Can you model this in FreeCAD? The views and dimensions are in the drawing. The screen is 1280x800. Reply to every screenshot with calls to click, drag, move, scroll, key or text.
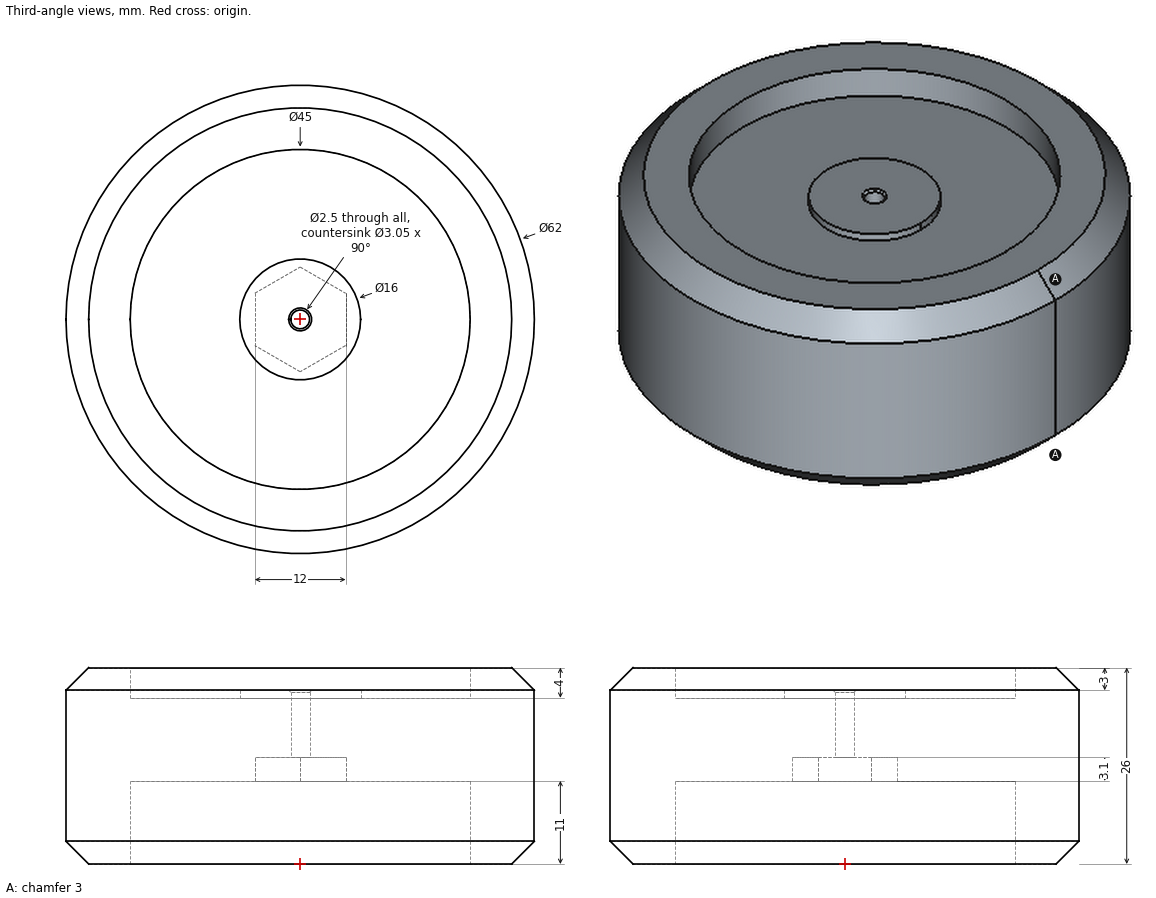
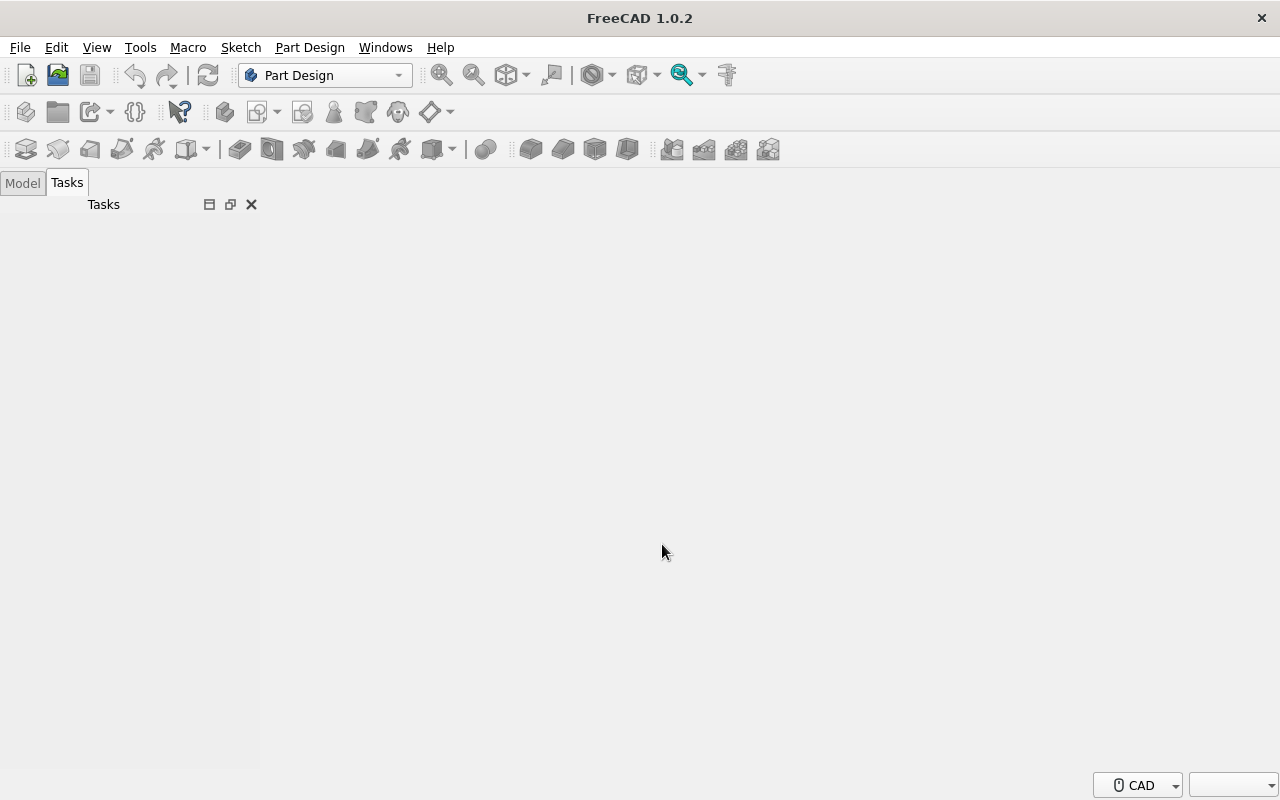
click(26, 76)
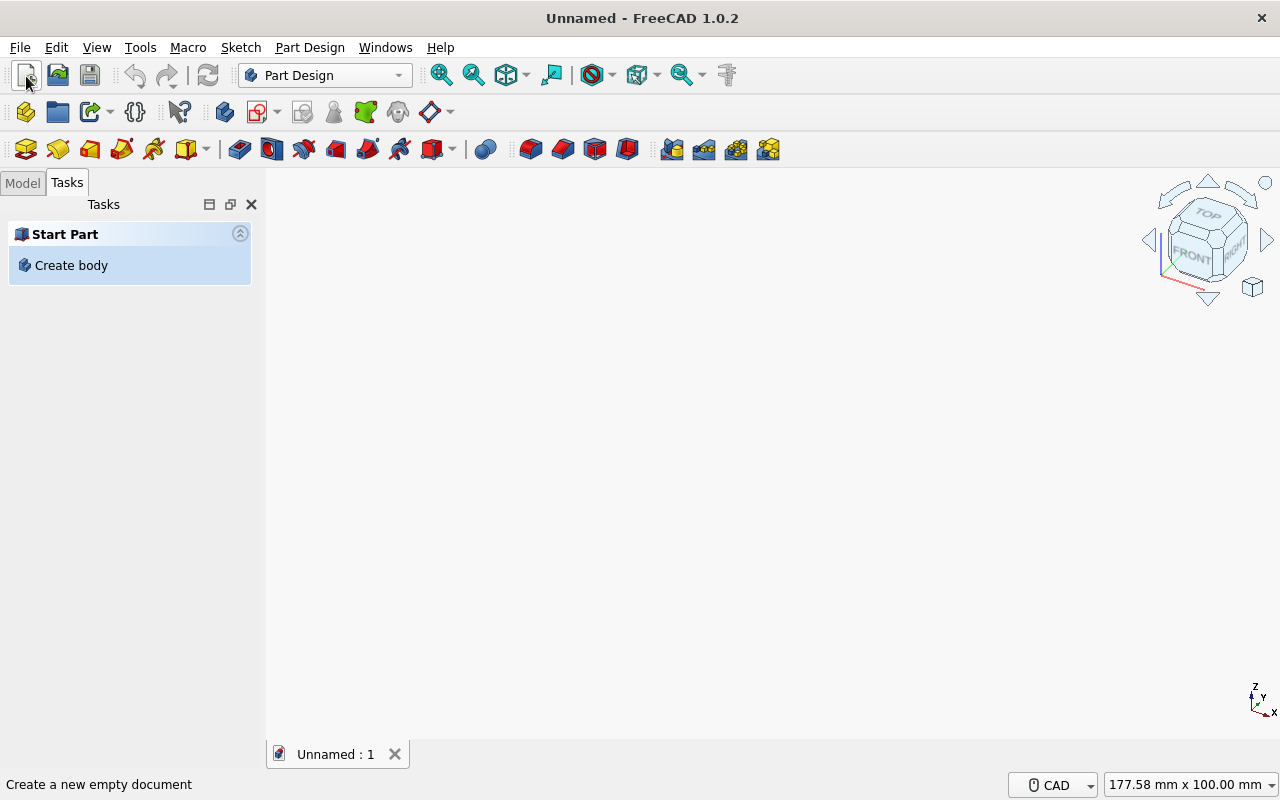
click(258, 112)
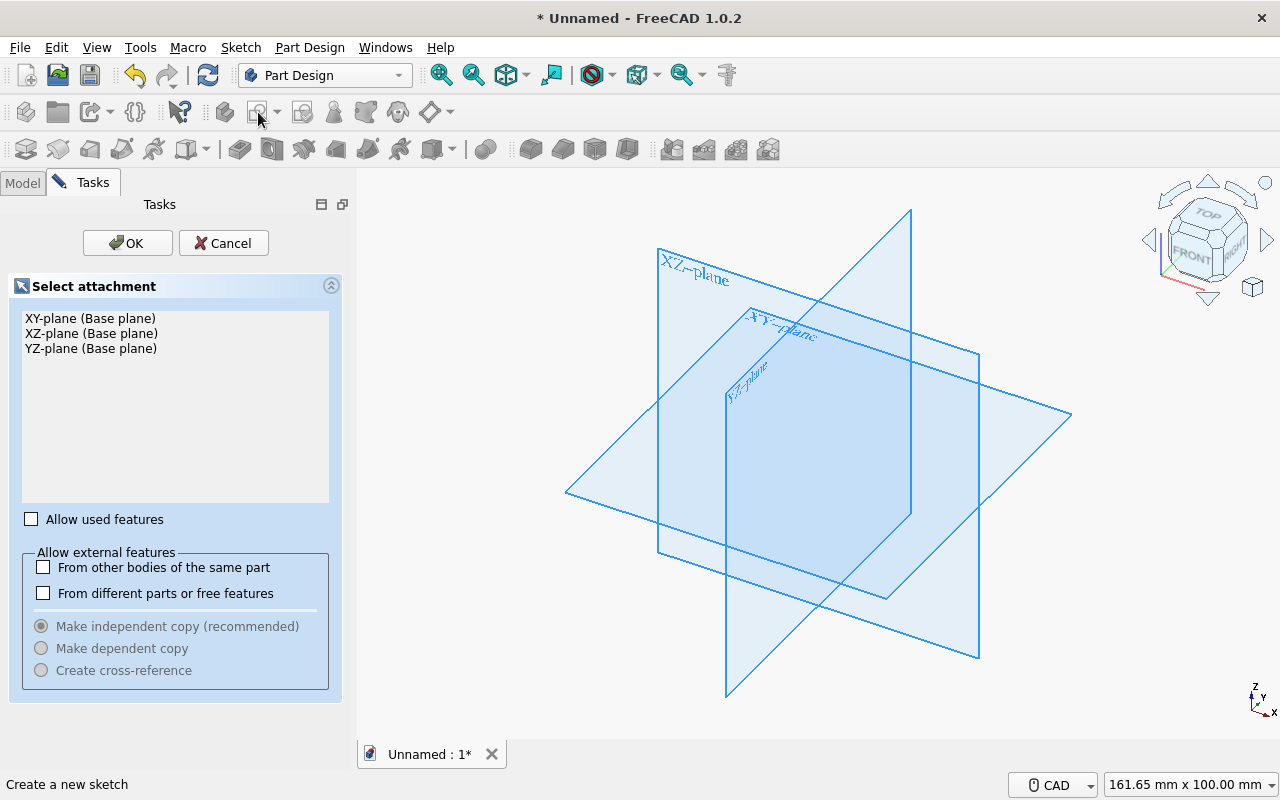
click(82, 318)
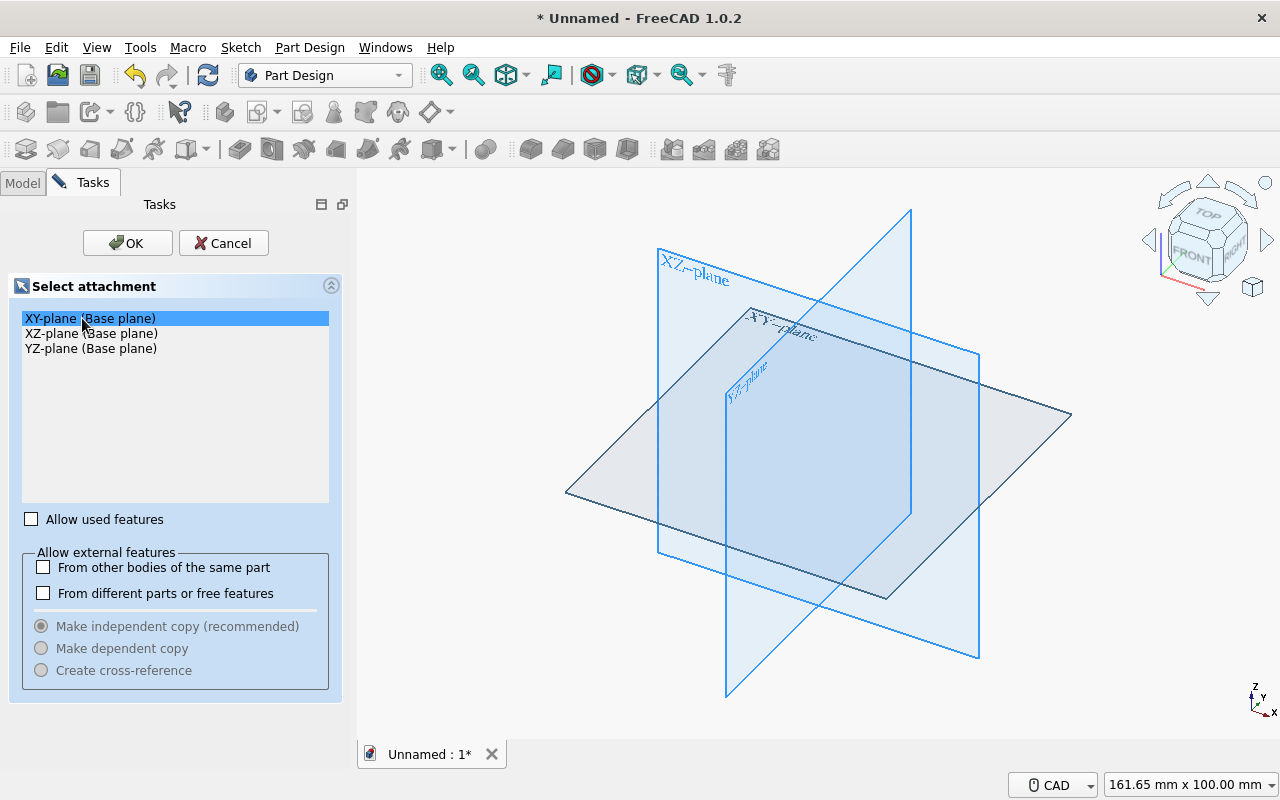
click(128, 243)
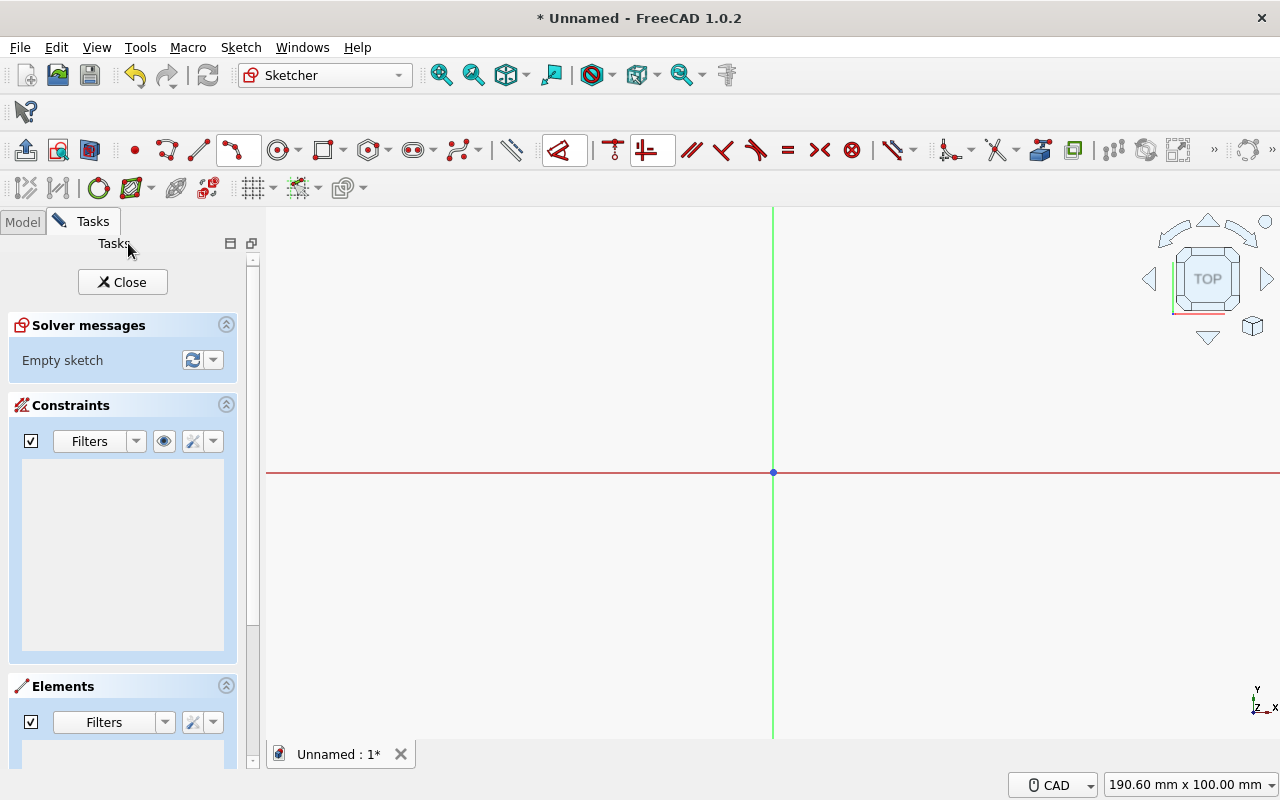
click(278, 150)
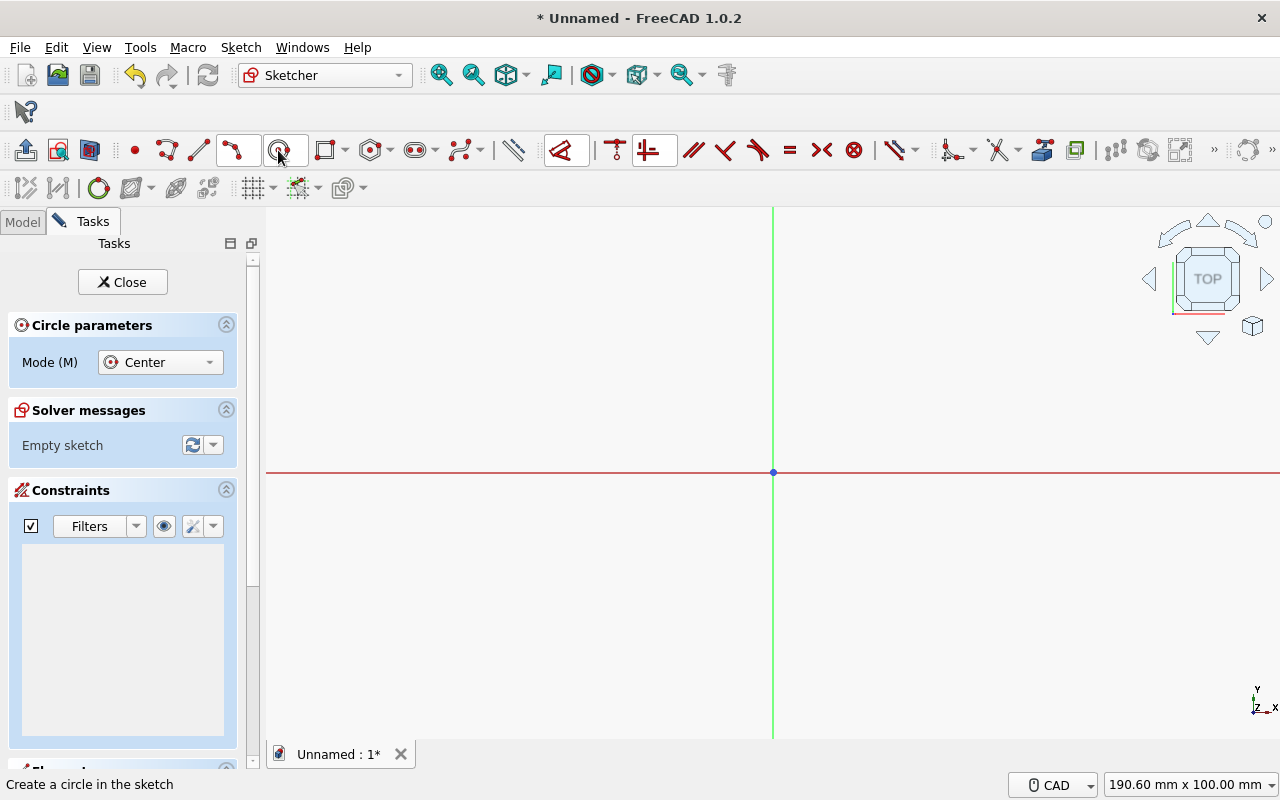
click(773, 473)
click(890, 356)
key(Escape)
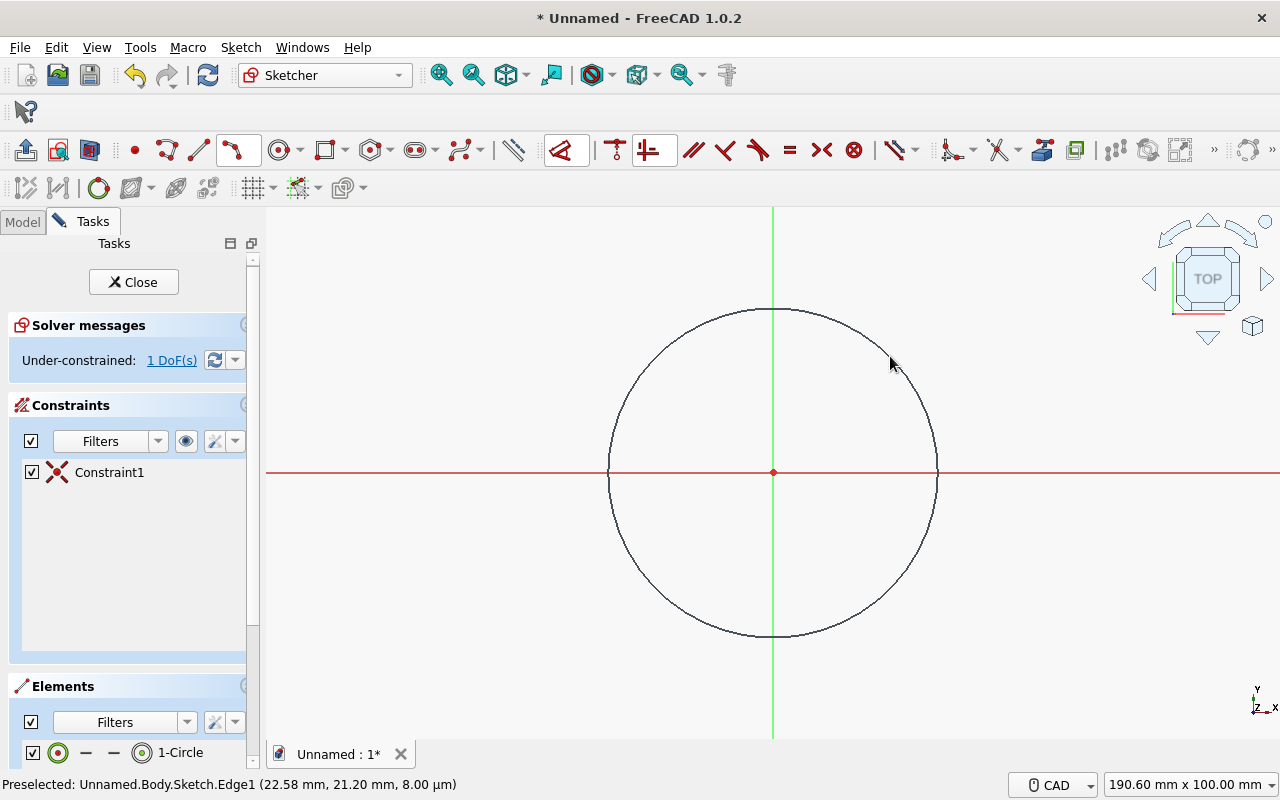
click(560, 150)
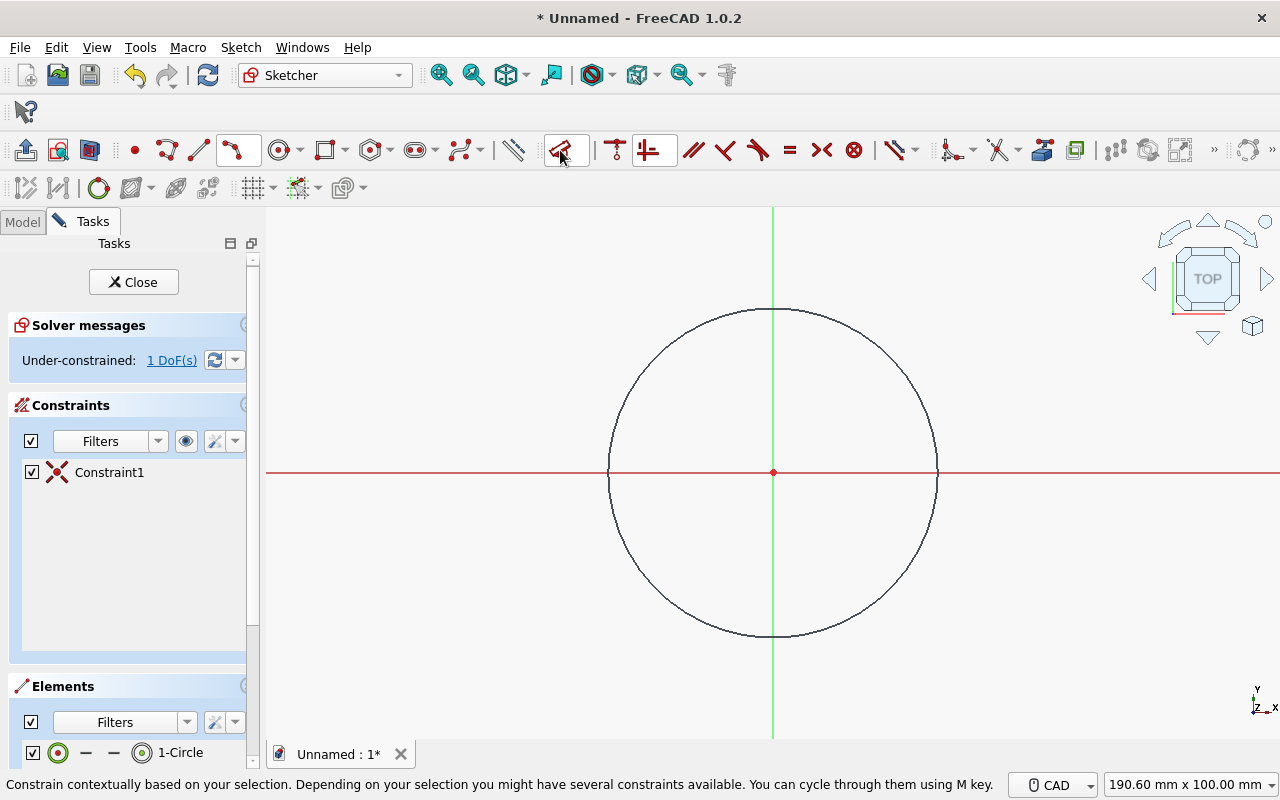
click(889, 356)
click(912, 333)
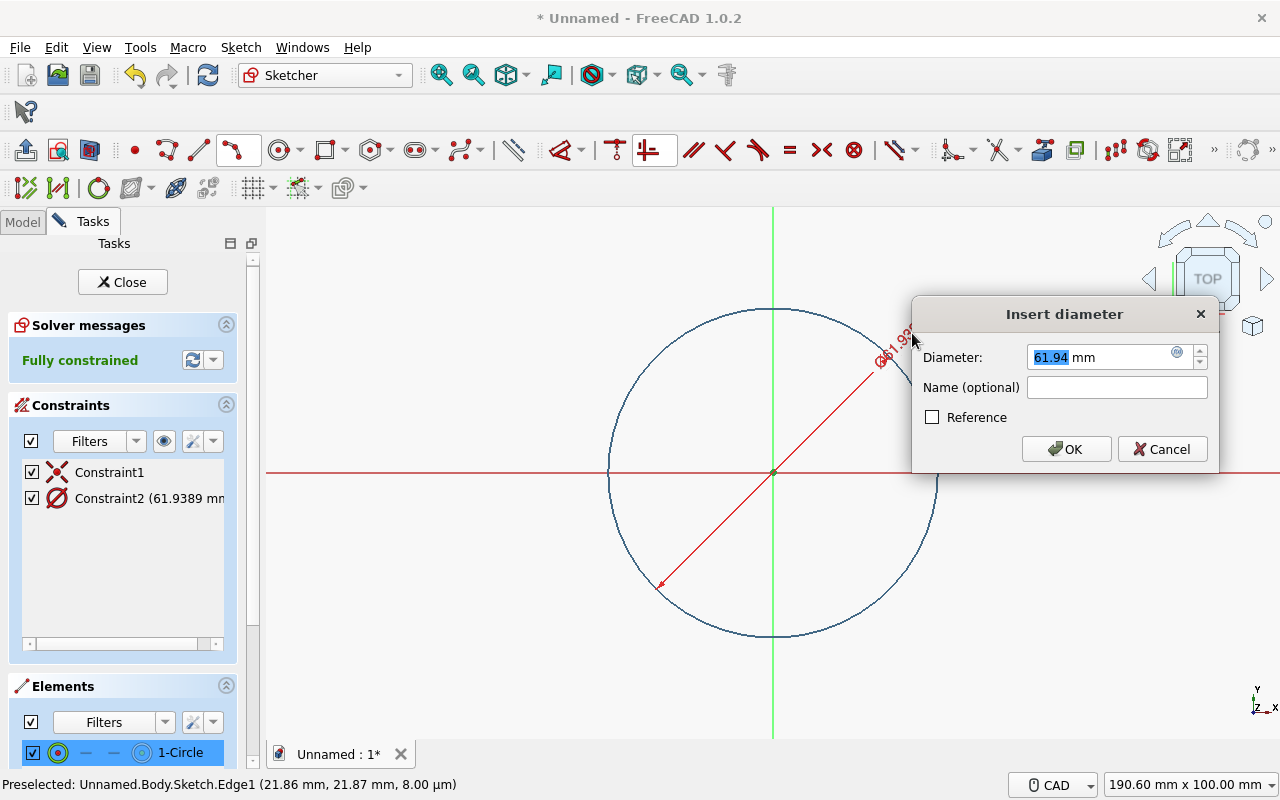
text(62)
key(Return)
key(Escape)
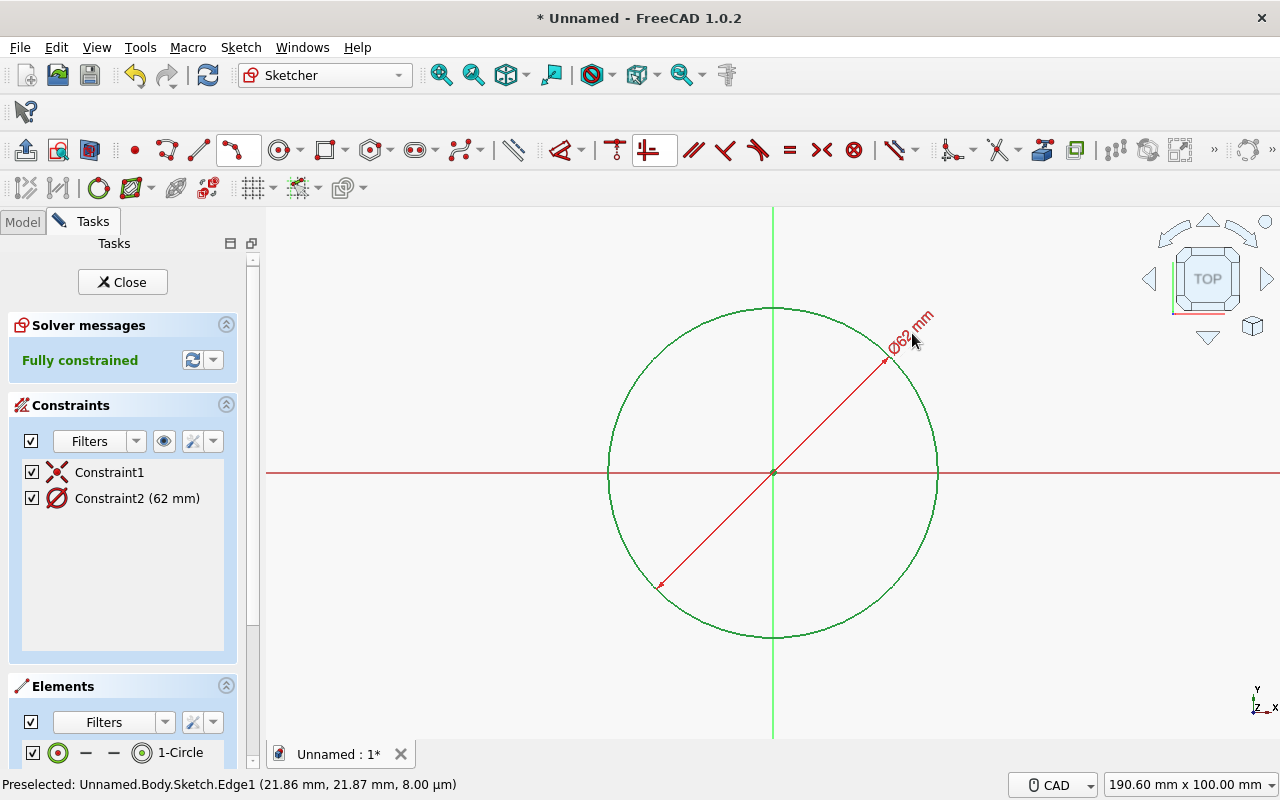
click(123, 282)